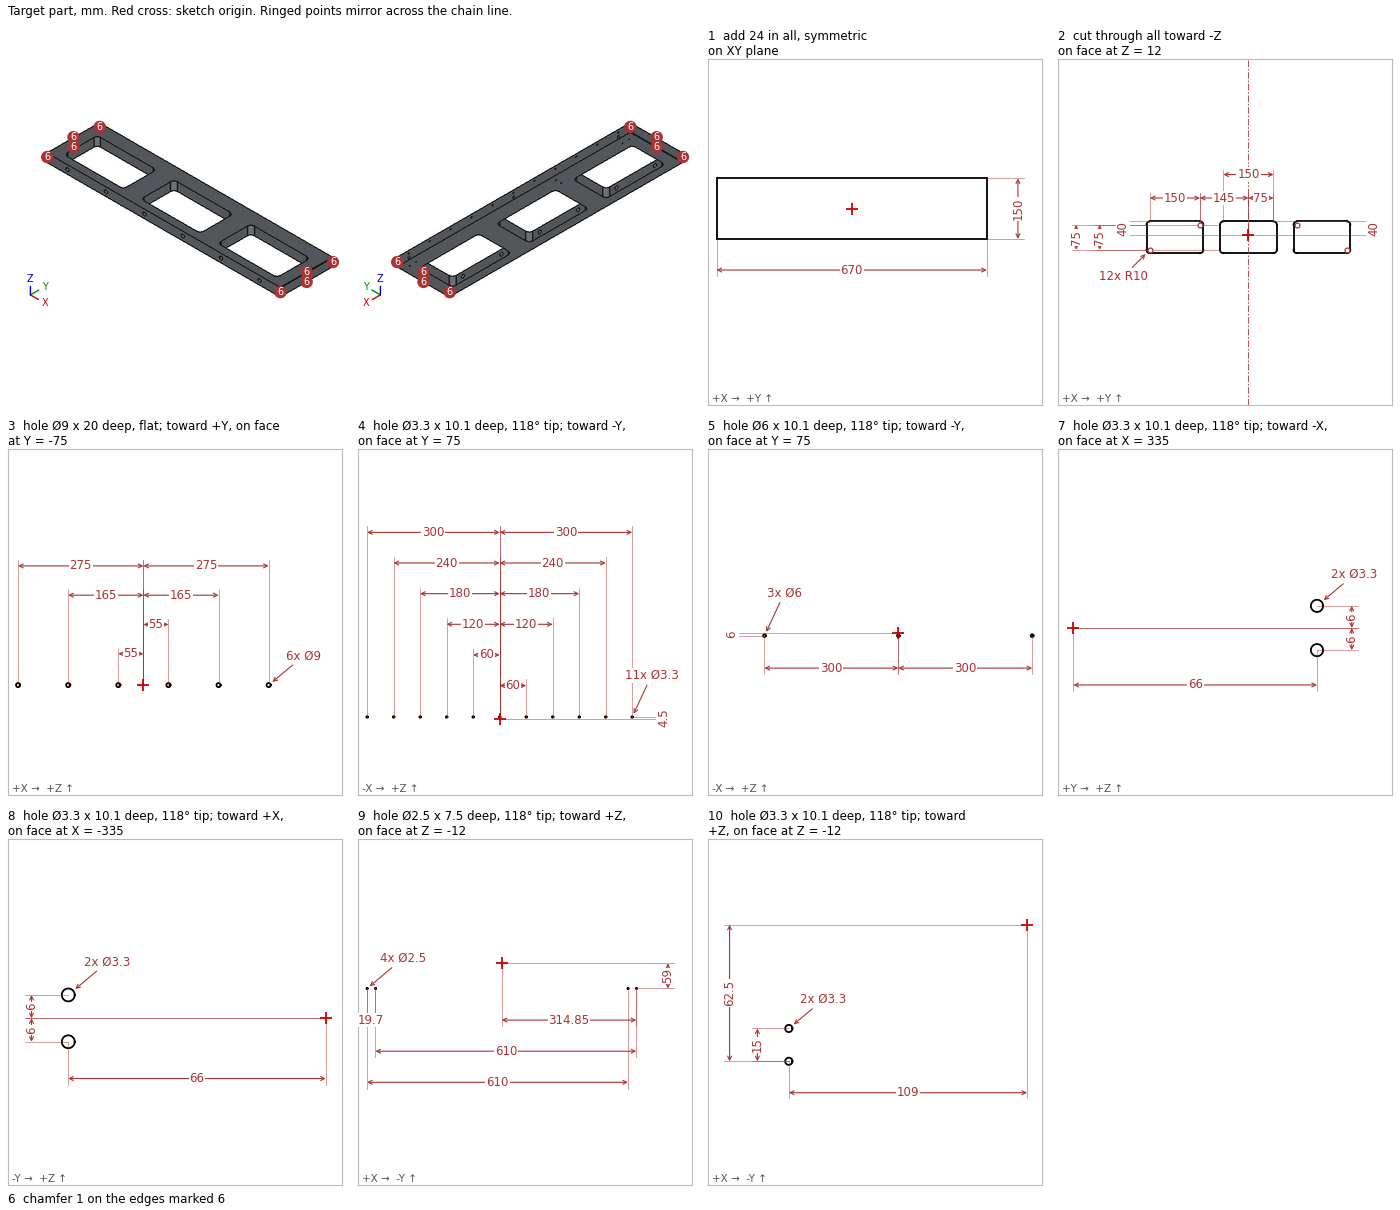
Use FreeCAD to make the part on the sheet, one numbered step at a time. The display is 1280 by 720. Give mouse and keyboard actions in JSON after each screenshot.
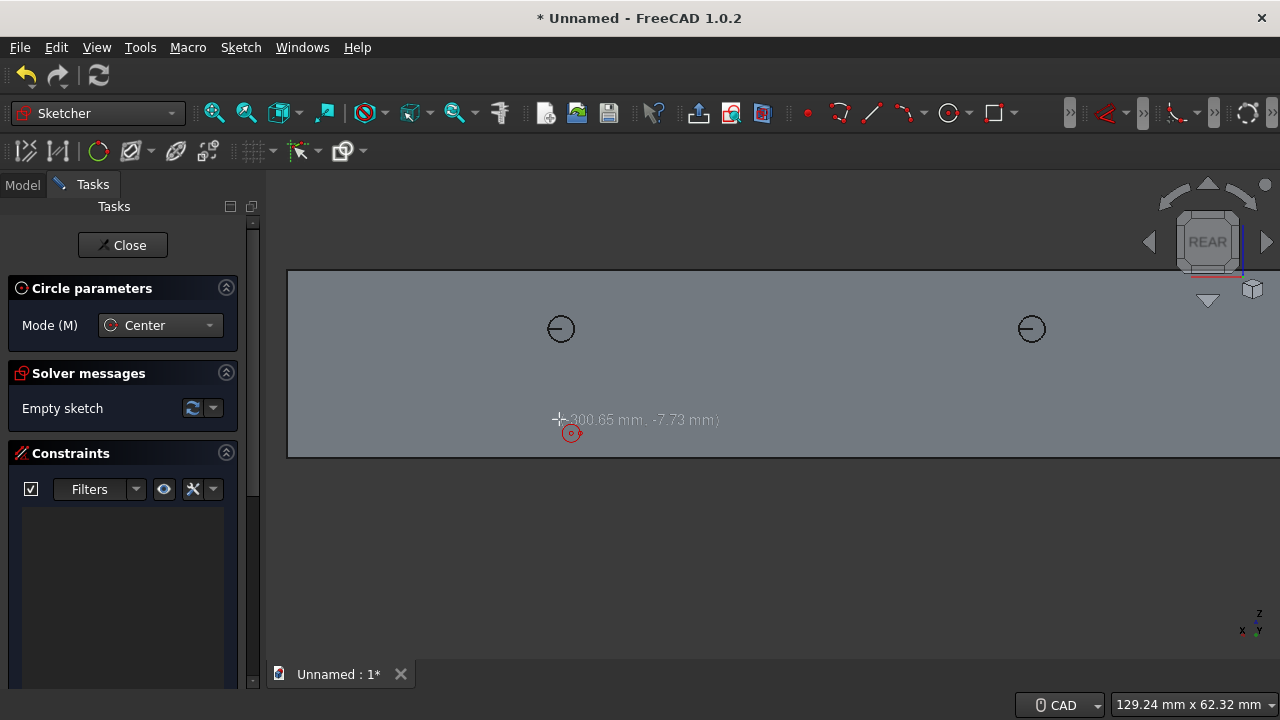
{"action": "scroll", "coordinate": [429, 416], "scroll_direction": "down", "scroll_amount": 11}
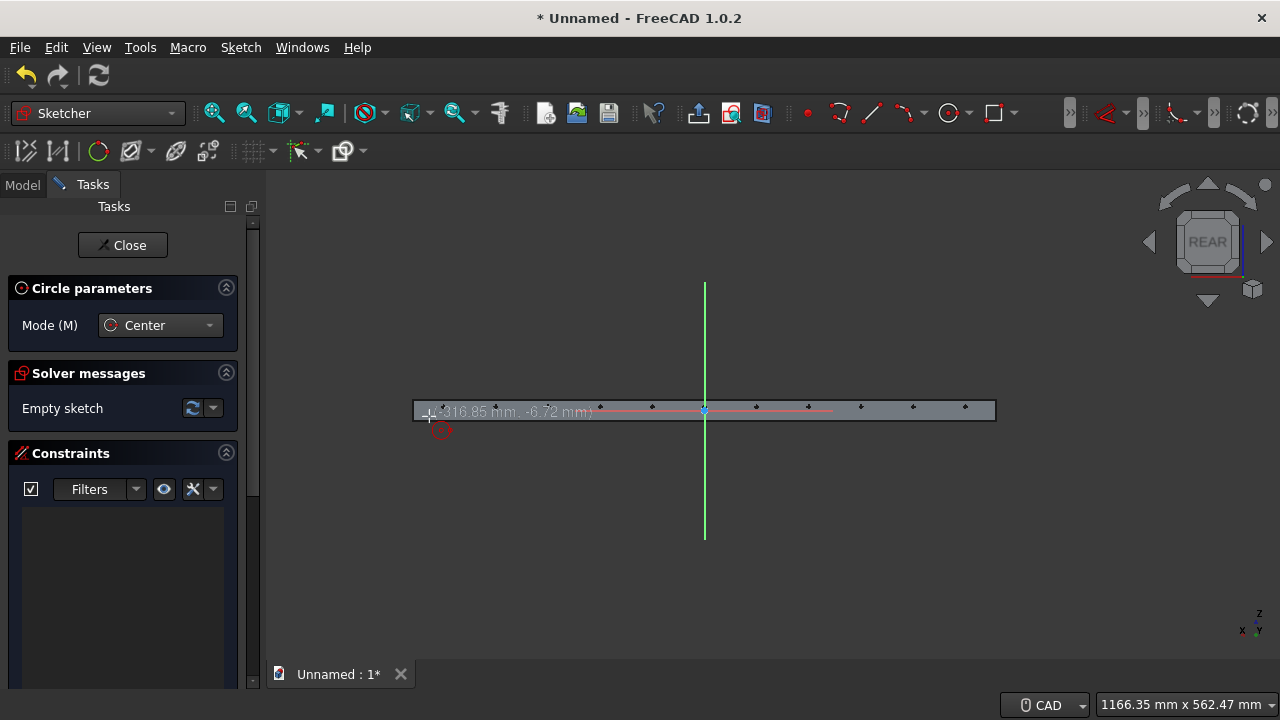
{"action": "scroll", "coordinate": [444, 416], "scroll_direction": "up", "scroll_amount": 6}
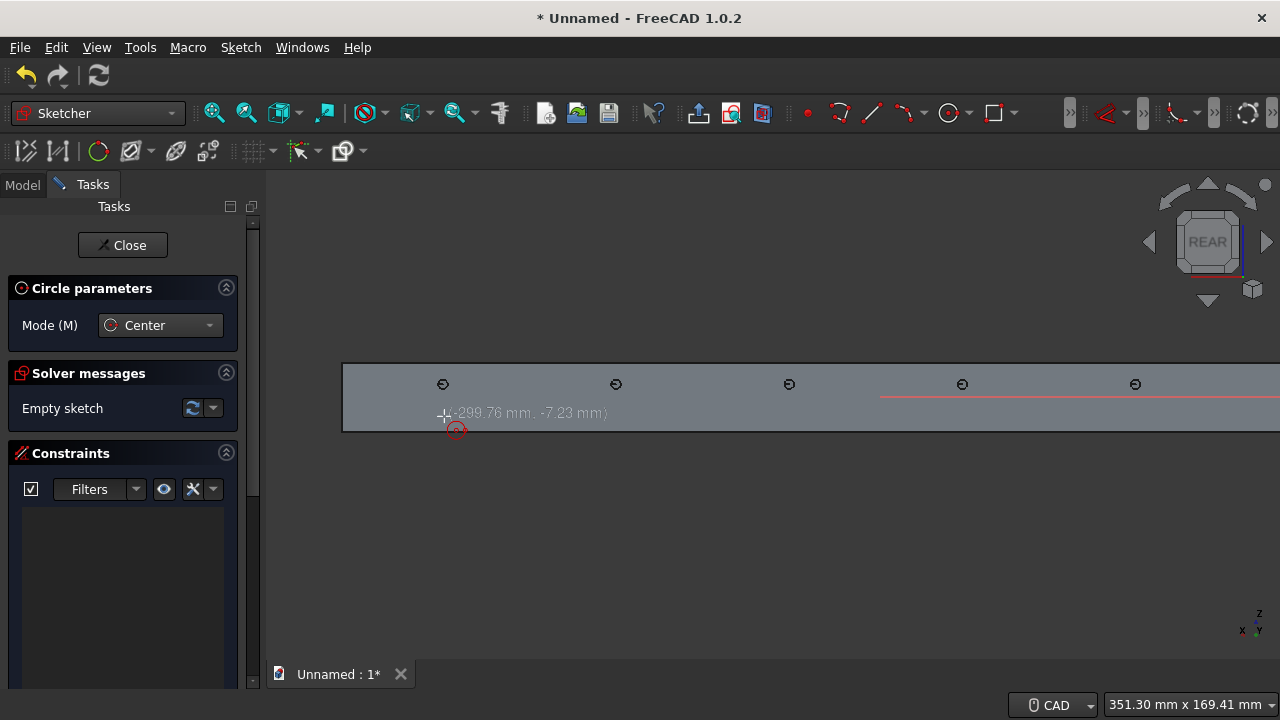
{"action": "left_click", "coordinate": [443, 415]}
{"action": "mouse_move", "coordinate": [449, 421]}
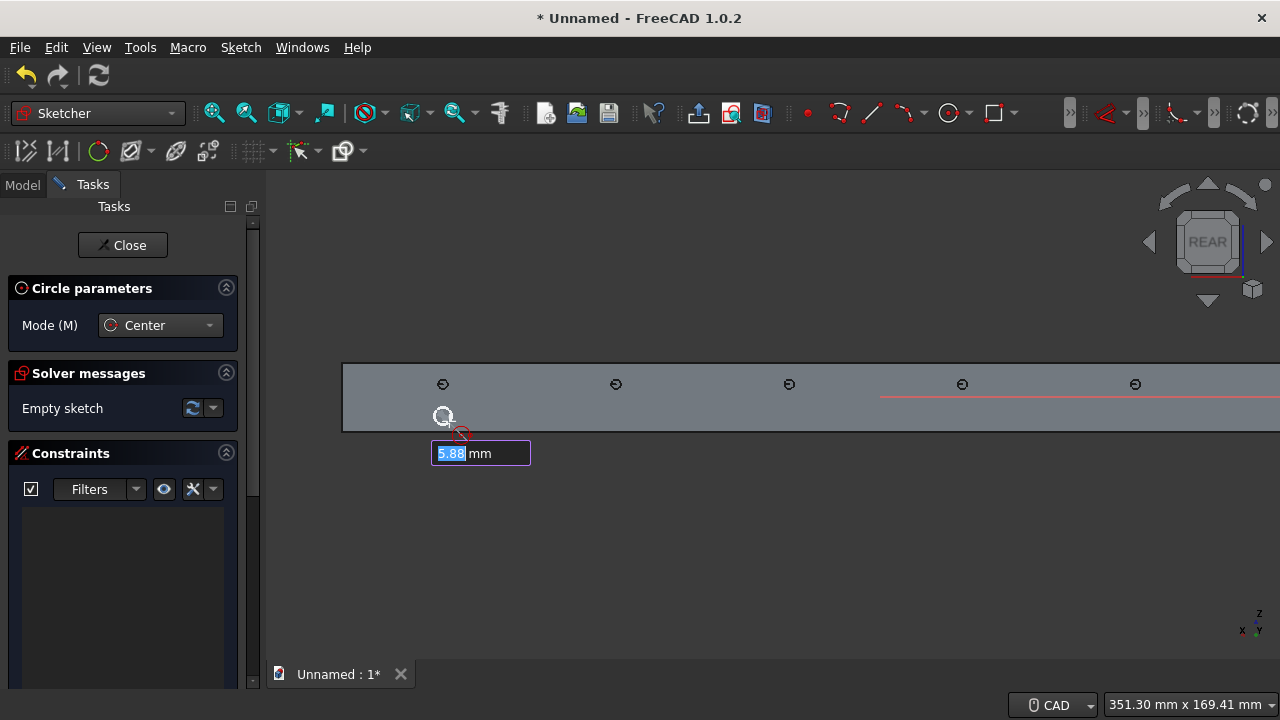
{"action": "type", "text": "6"}
{"action": "key", "text": "Return"}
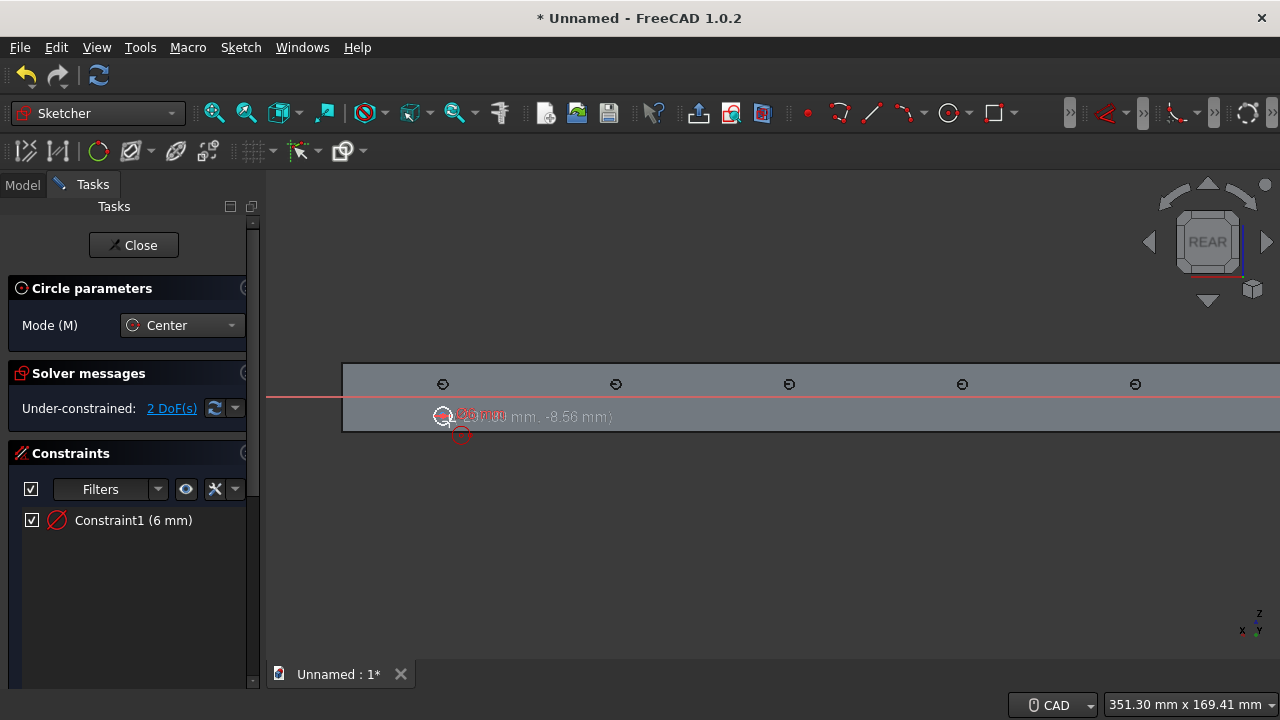
{"action": "scroll", "coordinate": [444, 416], "scroll_direction": "down", "scroll_amount": 6}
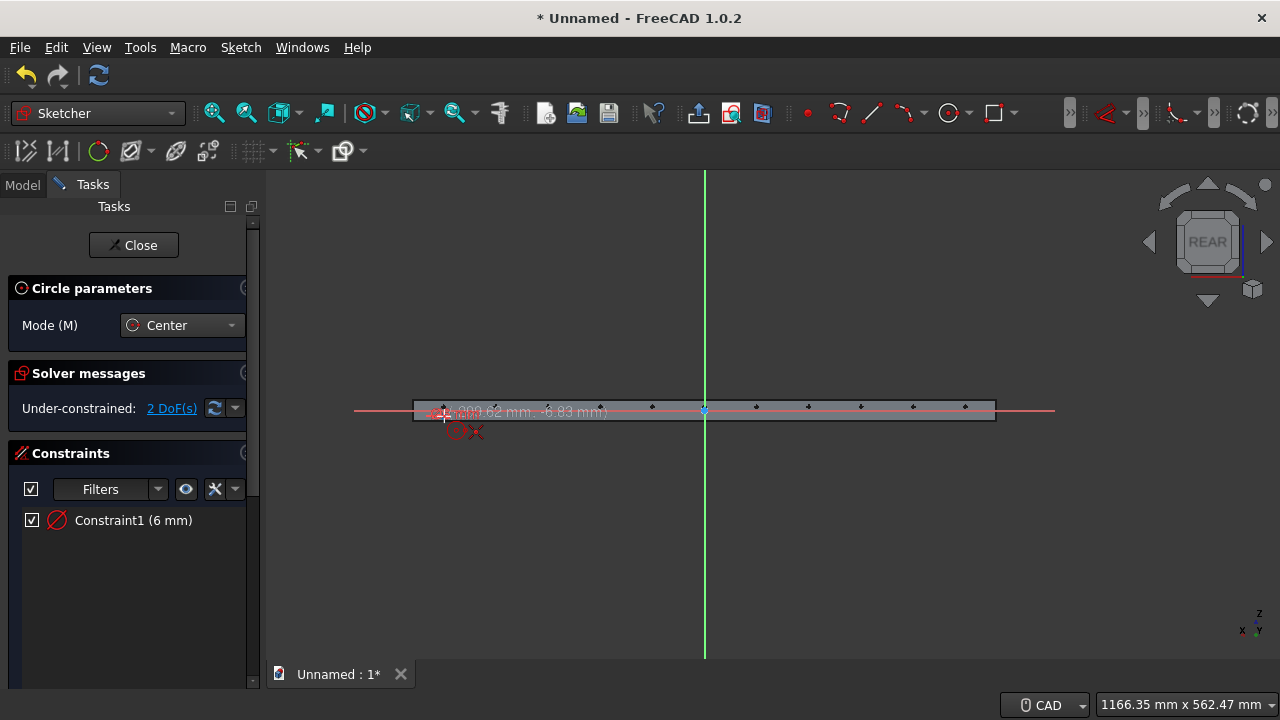
{"action": "scroll", "coordinate": [965, 416], "scroll_direction": "up", "scroll_amount": 11}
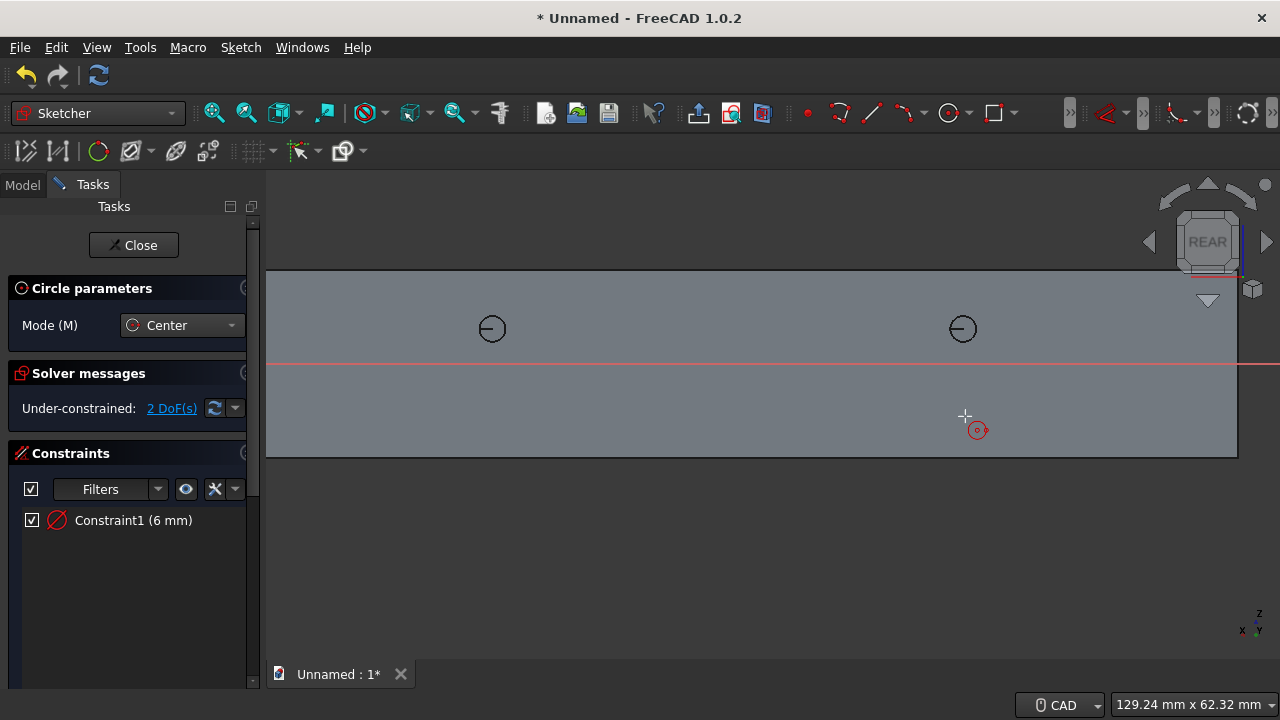
{"action": "scroll", "coordinate": [966, 416], "scroll_direction": "down", "scroll_amount": 11}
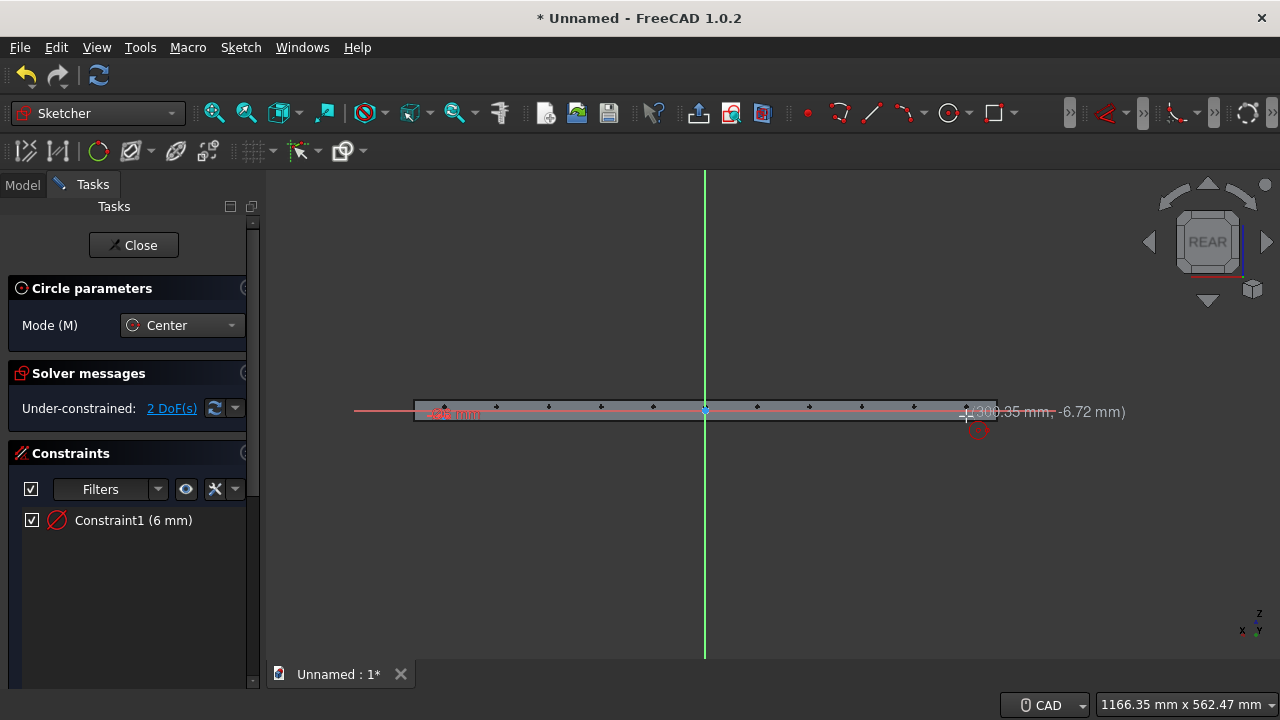
{"action": "scroll", "coordinate": [966, 416], "scroll_direction": "up", "scroll_amount": 6}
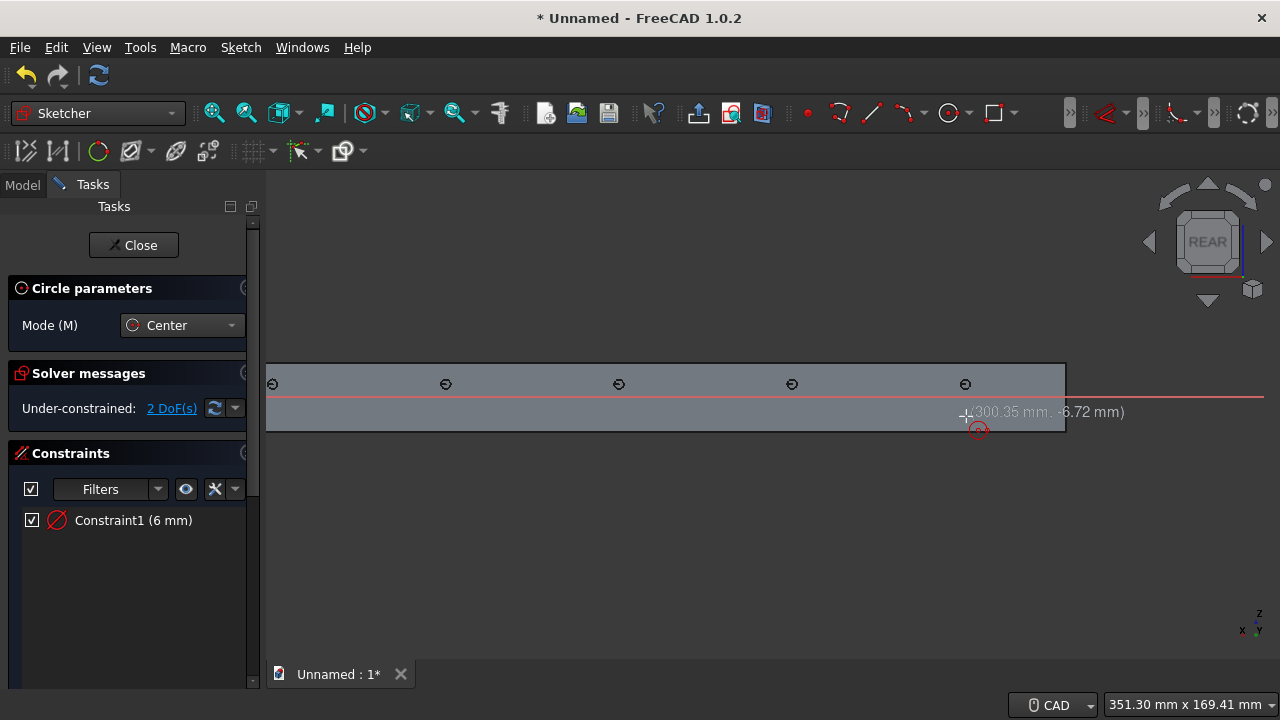
{"action": "left_click", "coordinate": [965, 415]}
{"action": "mouse_move", "coordinate": [972, 421]}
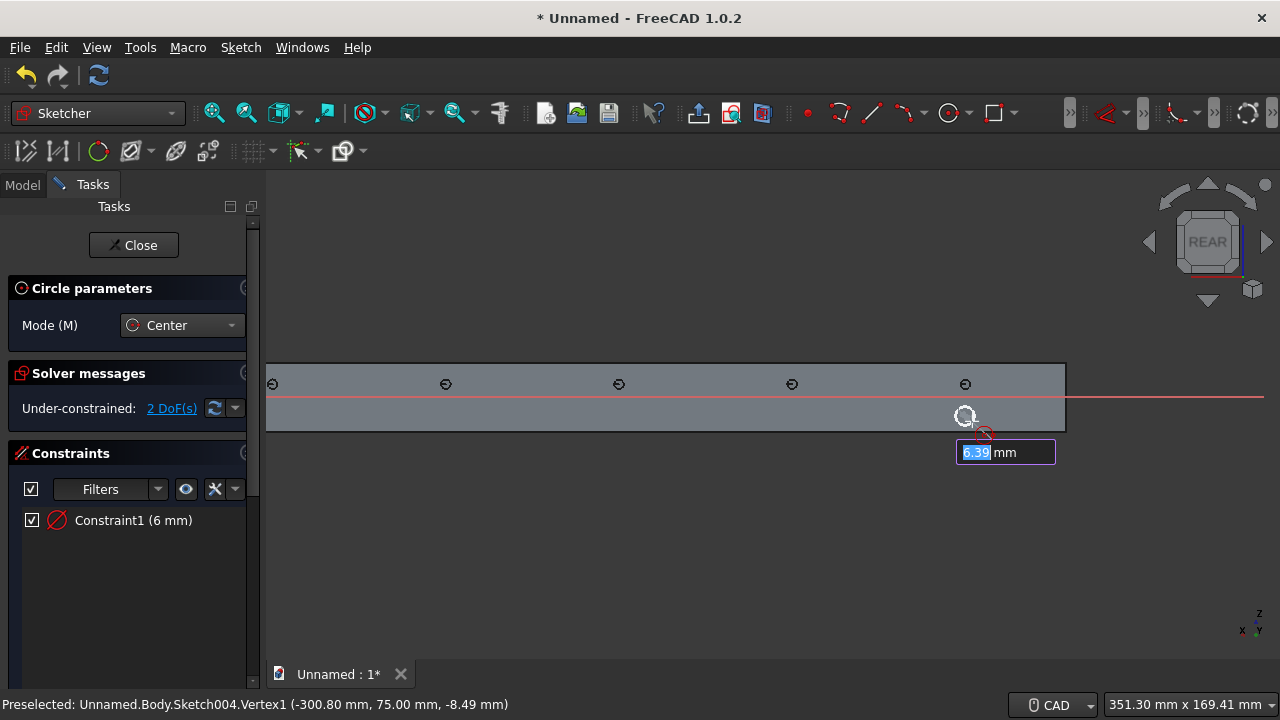
{"action": "type", "text": "6"}
{"action": "key", "text": "Return"}